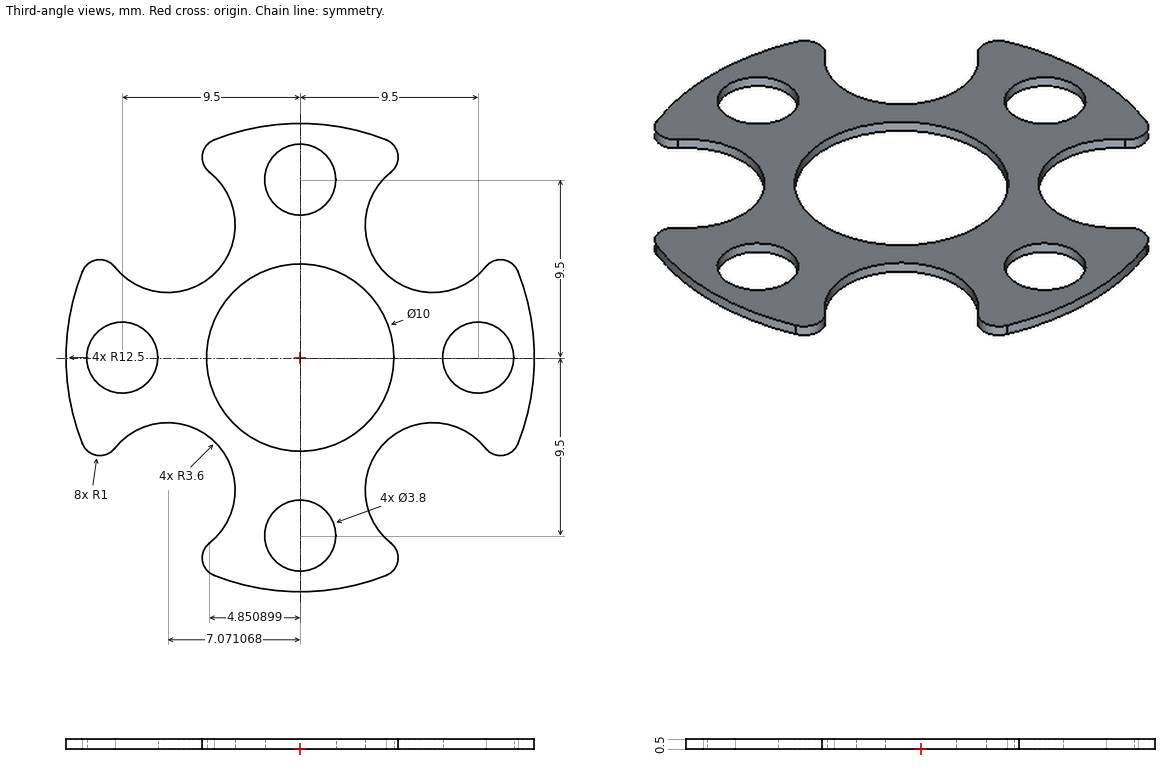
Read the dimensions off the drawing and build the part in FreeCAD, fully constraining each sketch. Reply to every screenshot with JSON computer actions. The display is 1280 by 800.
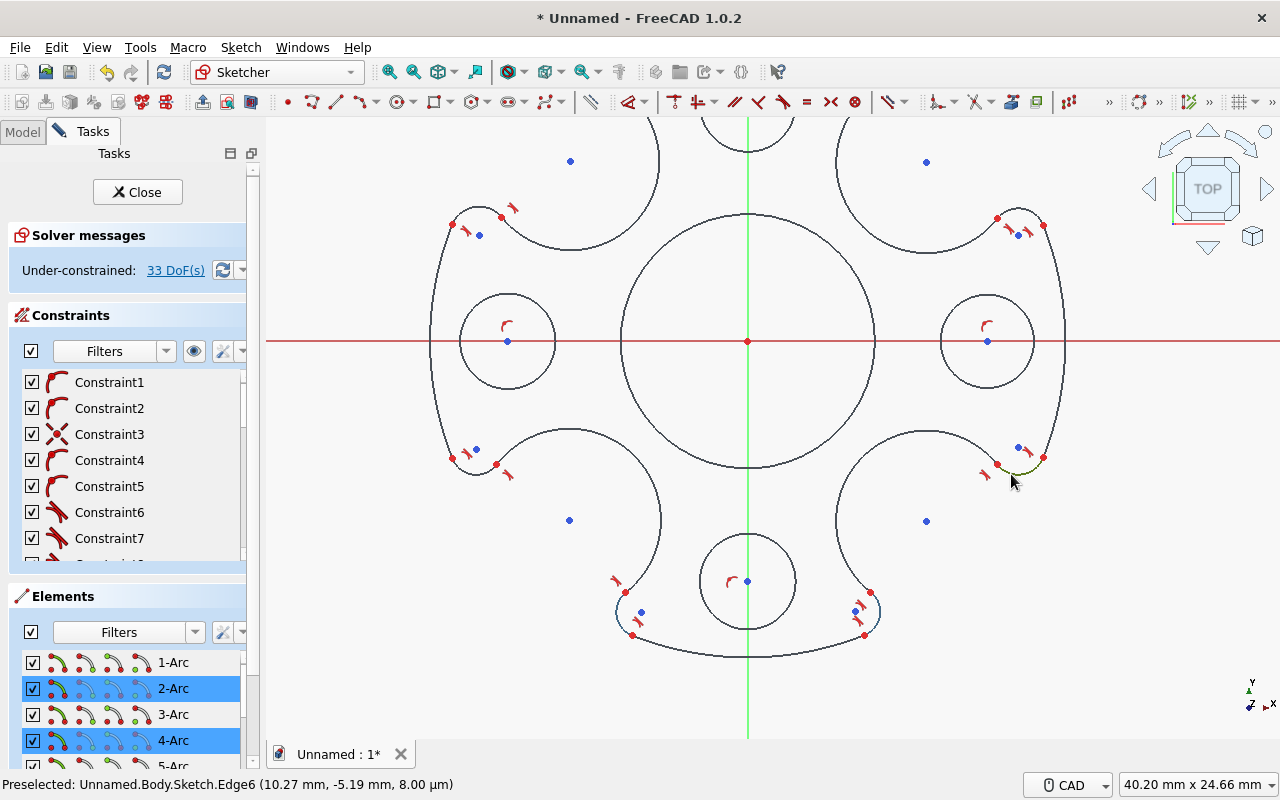
{"action": "left_click", "coordinate": [1033, 213]}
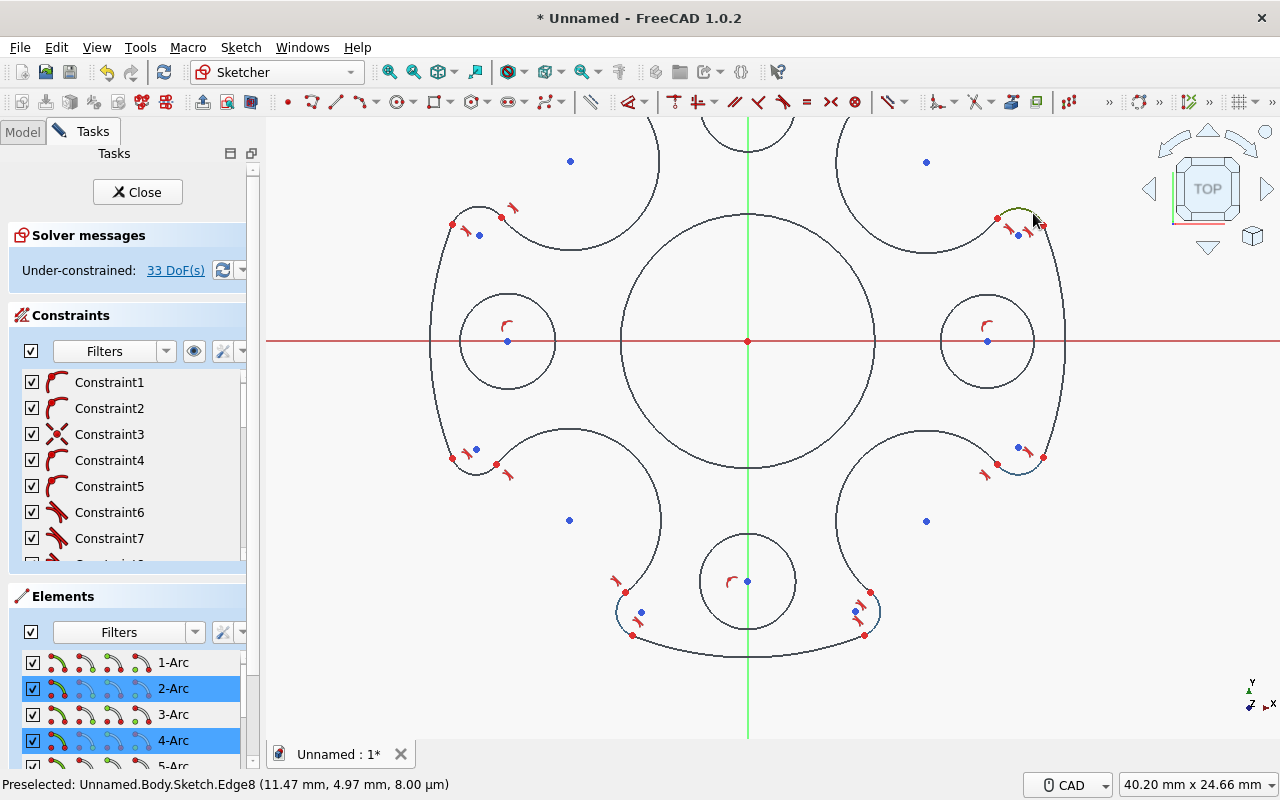
{"action": "scroll", "coordinate": [617, 604], "scroll_direction": "down", "scroll_amount": 2}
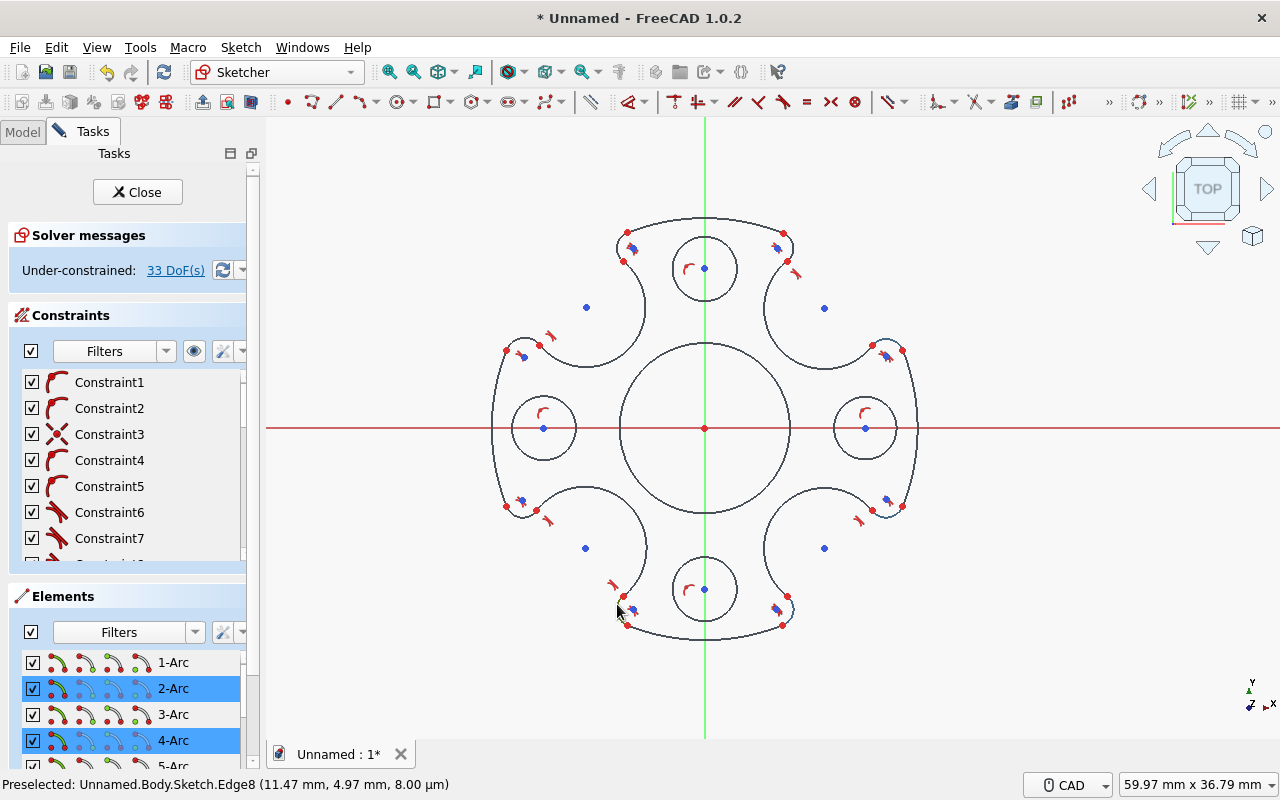
{"action": "scroll", "coordinate": [793, 253], "scroll_direction": "up", "scroll_amount": 2}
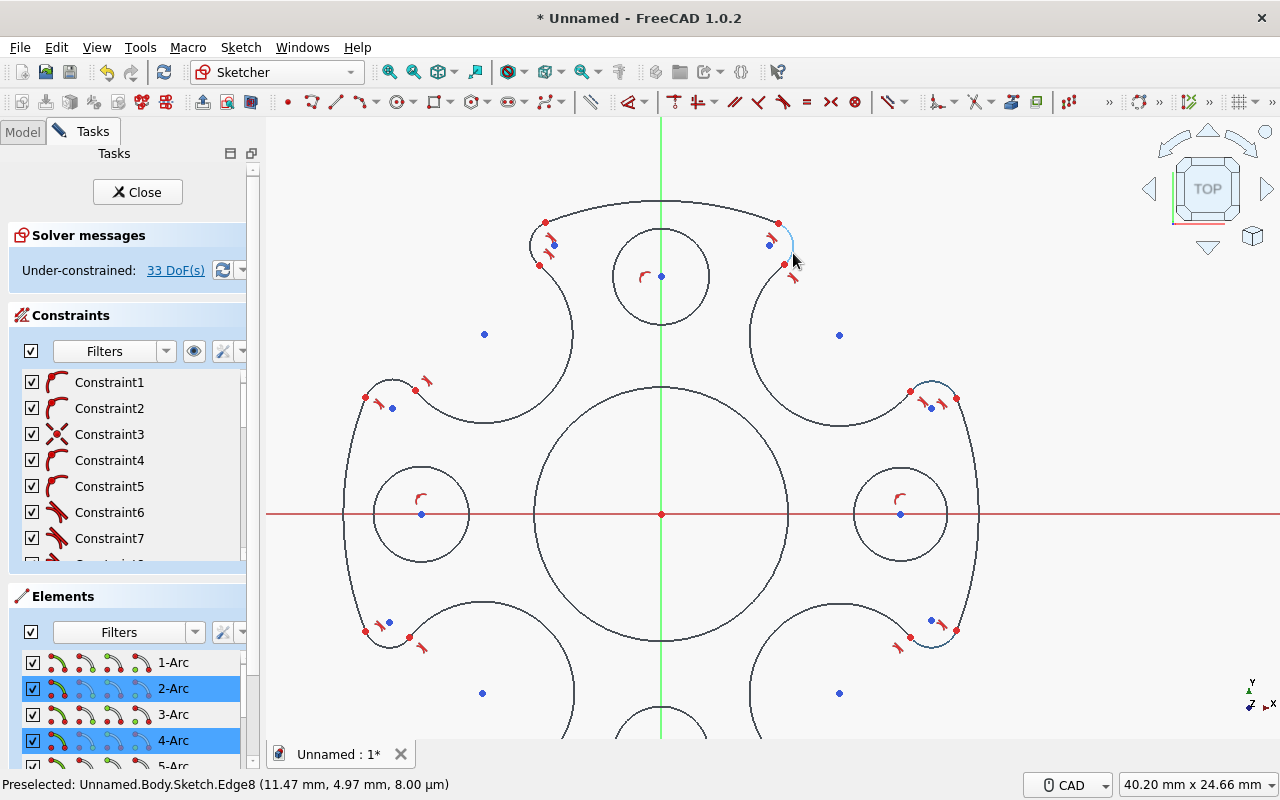
{"action": "left_click", "coordinate": [792, 253]}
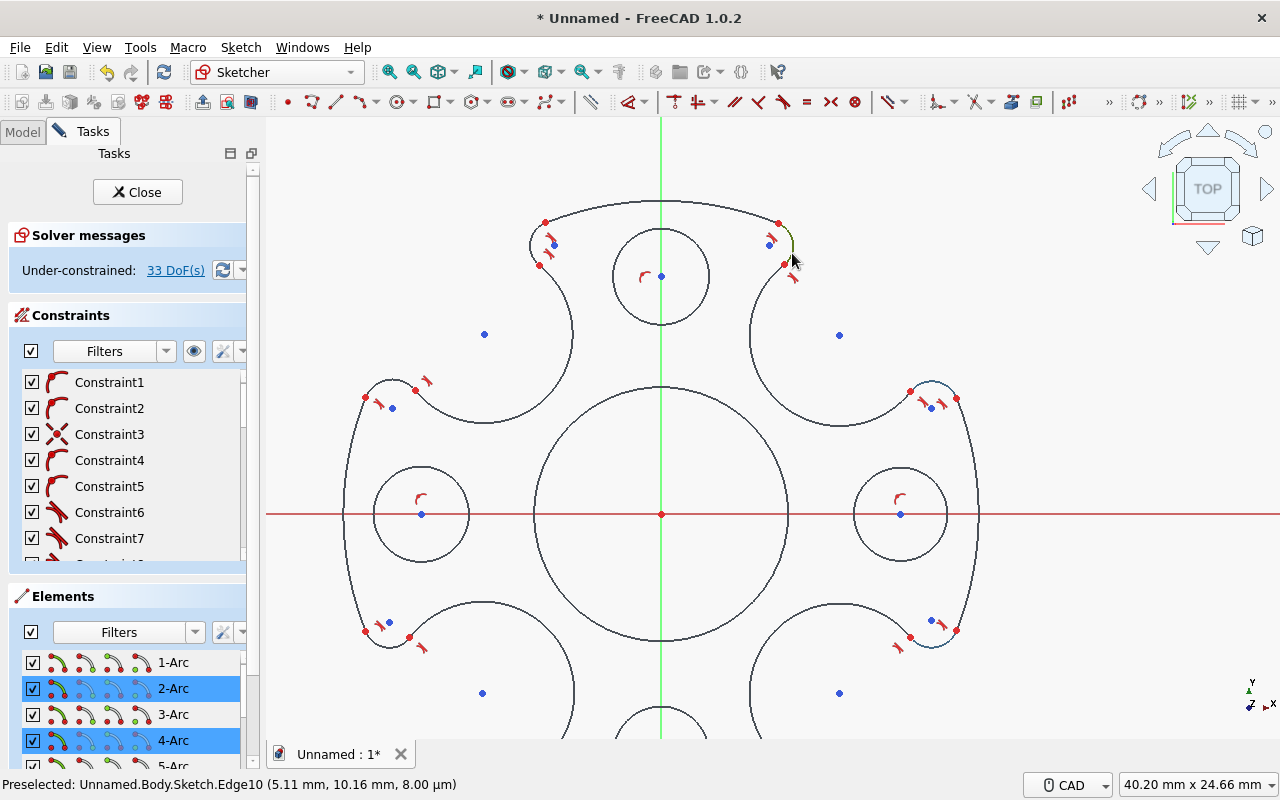
{"action": "left_click", "coordinate": [534, 233]}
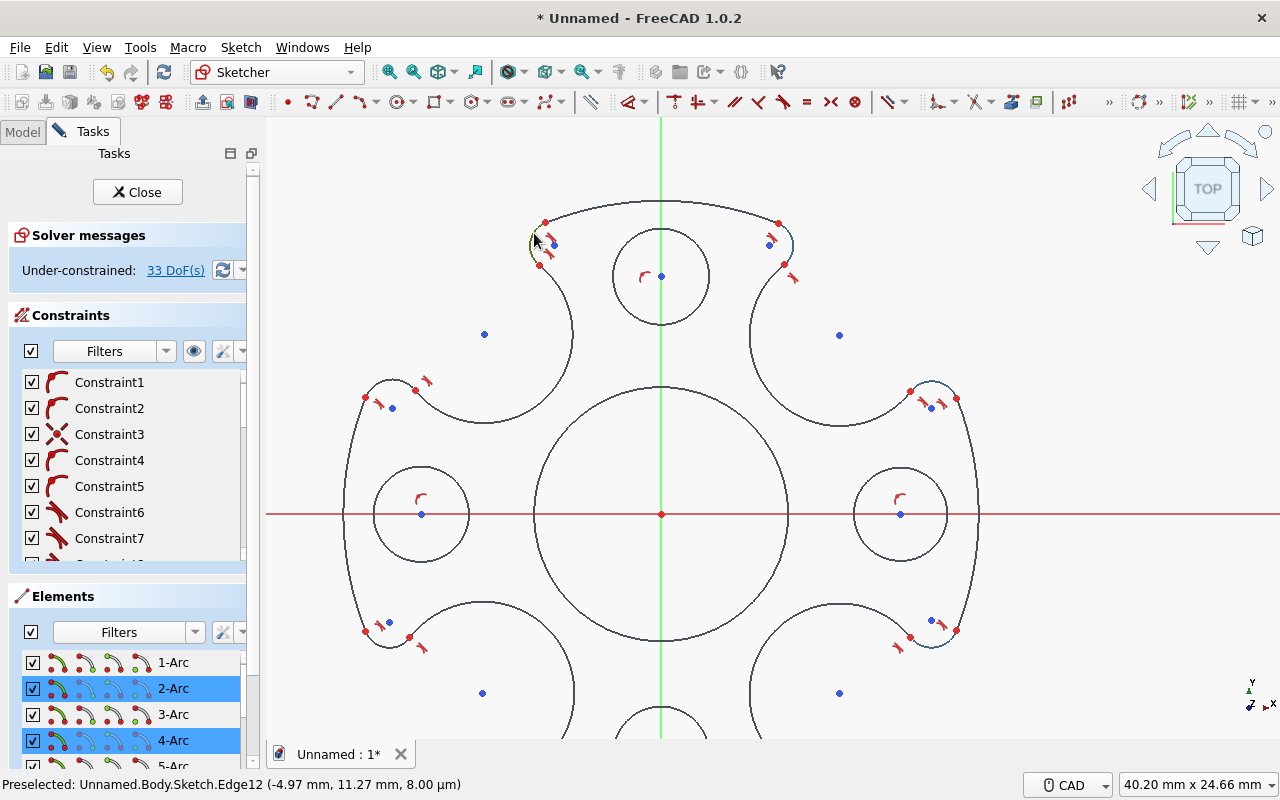
{"action": "left_click", "coordinate": [400, 381]}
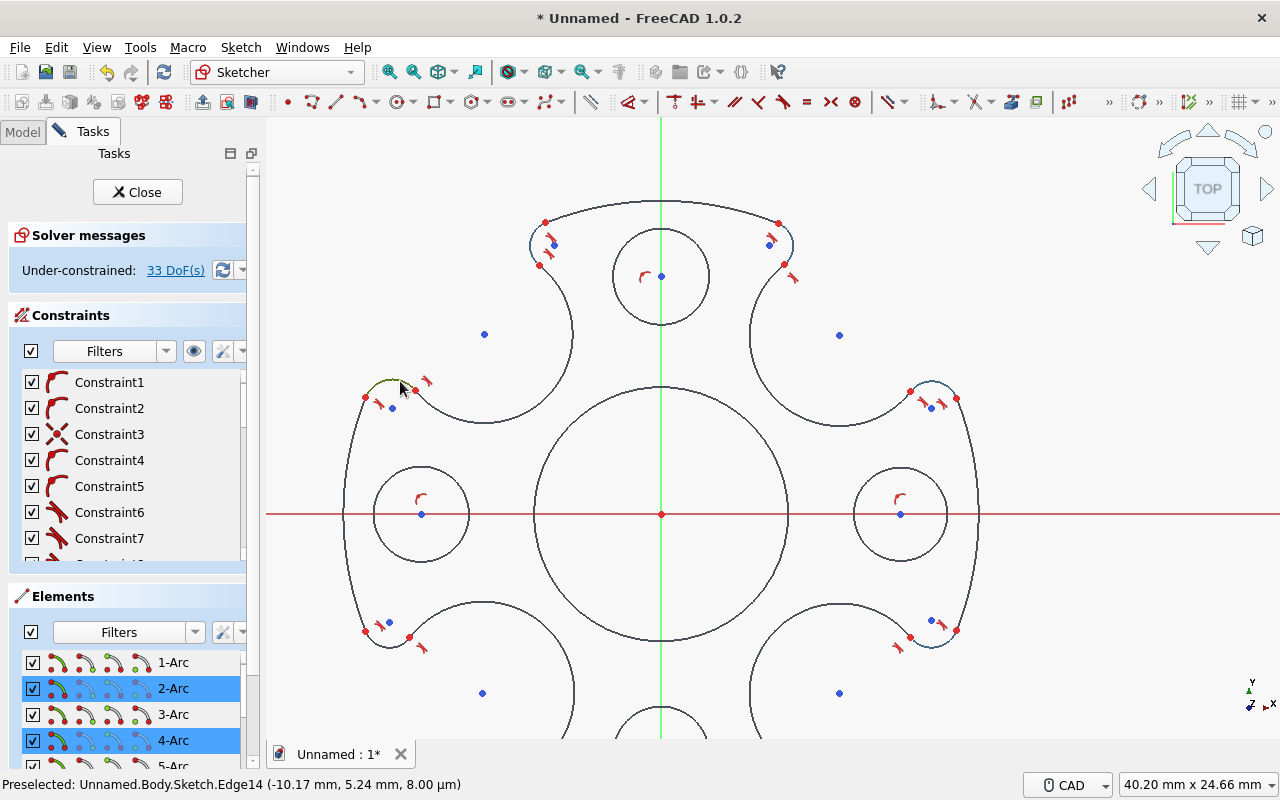
{"action": "left_click", "coordinate": [376, 644]}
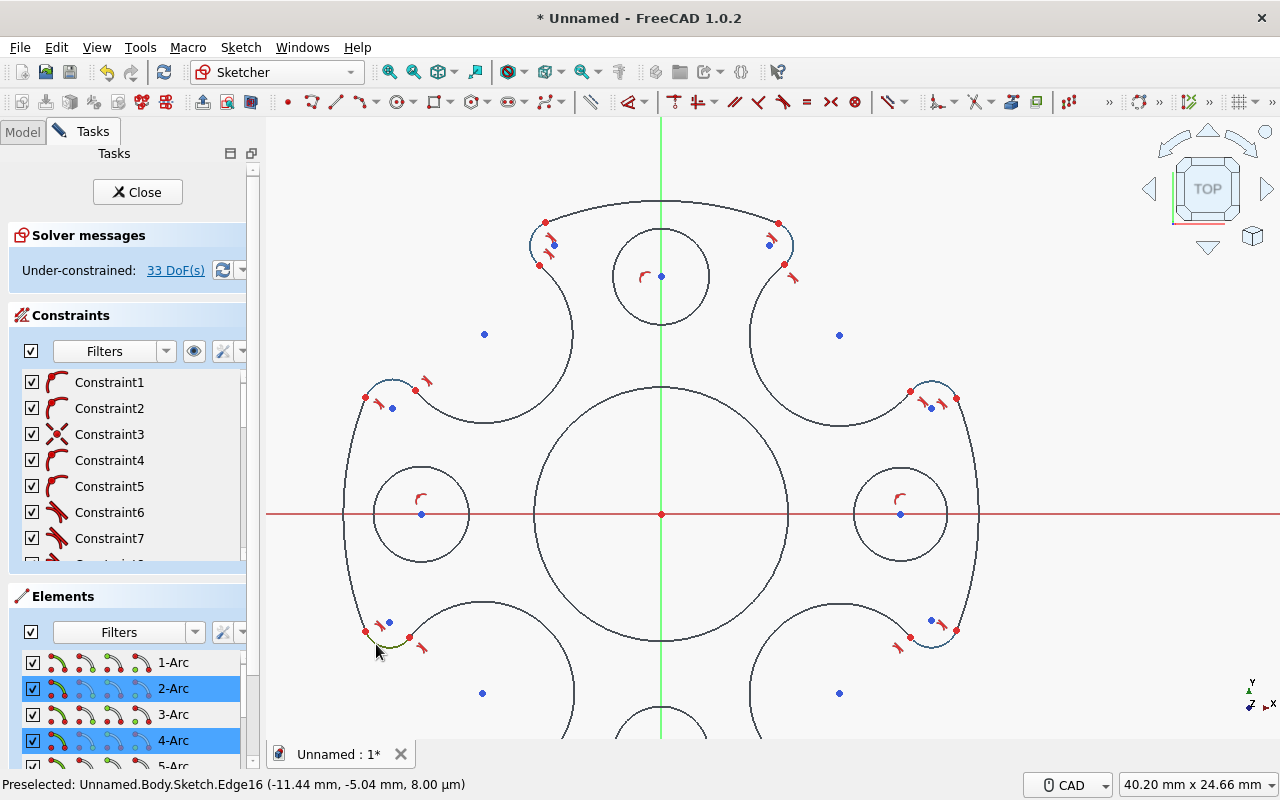
{"action": "key", "text": "e"}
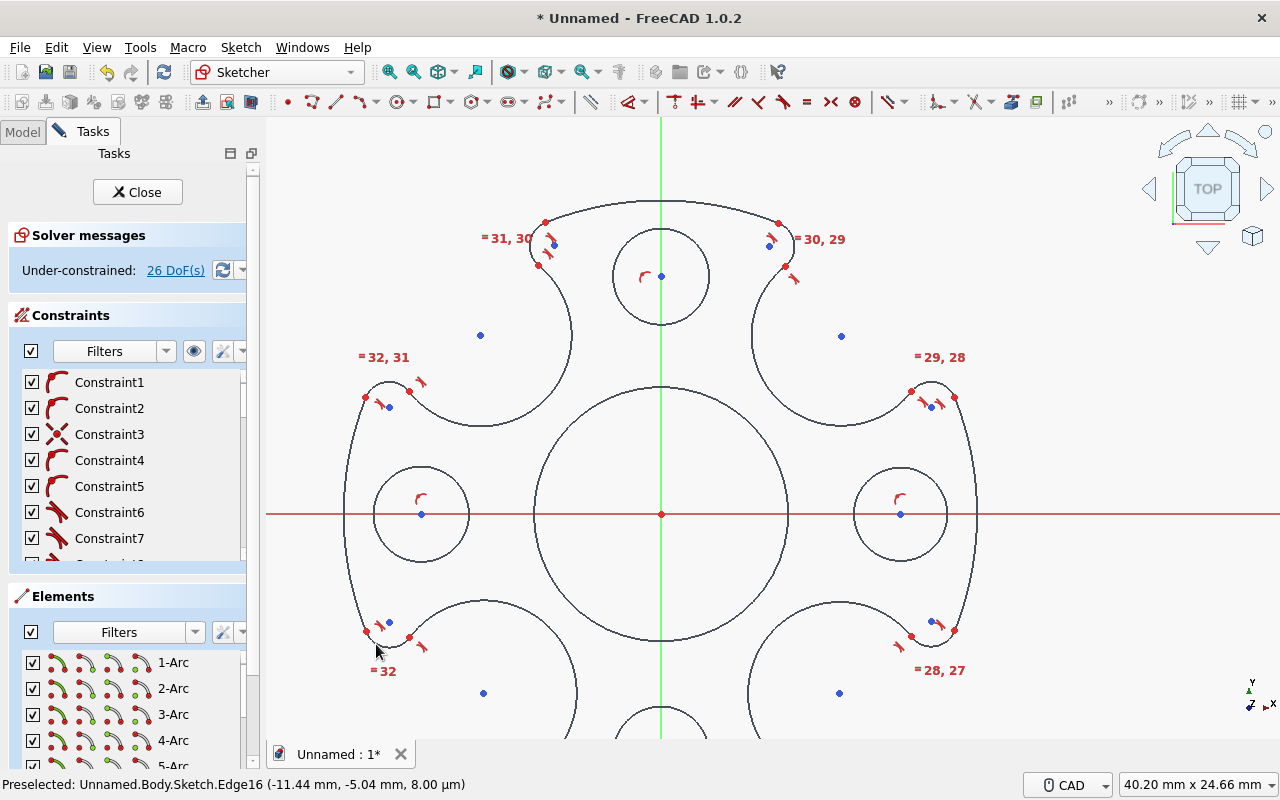
{"action": "left_click", "coordinate": [576, 683]}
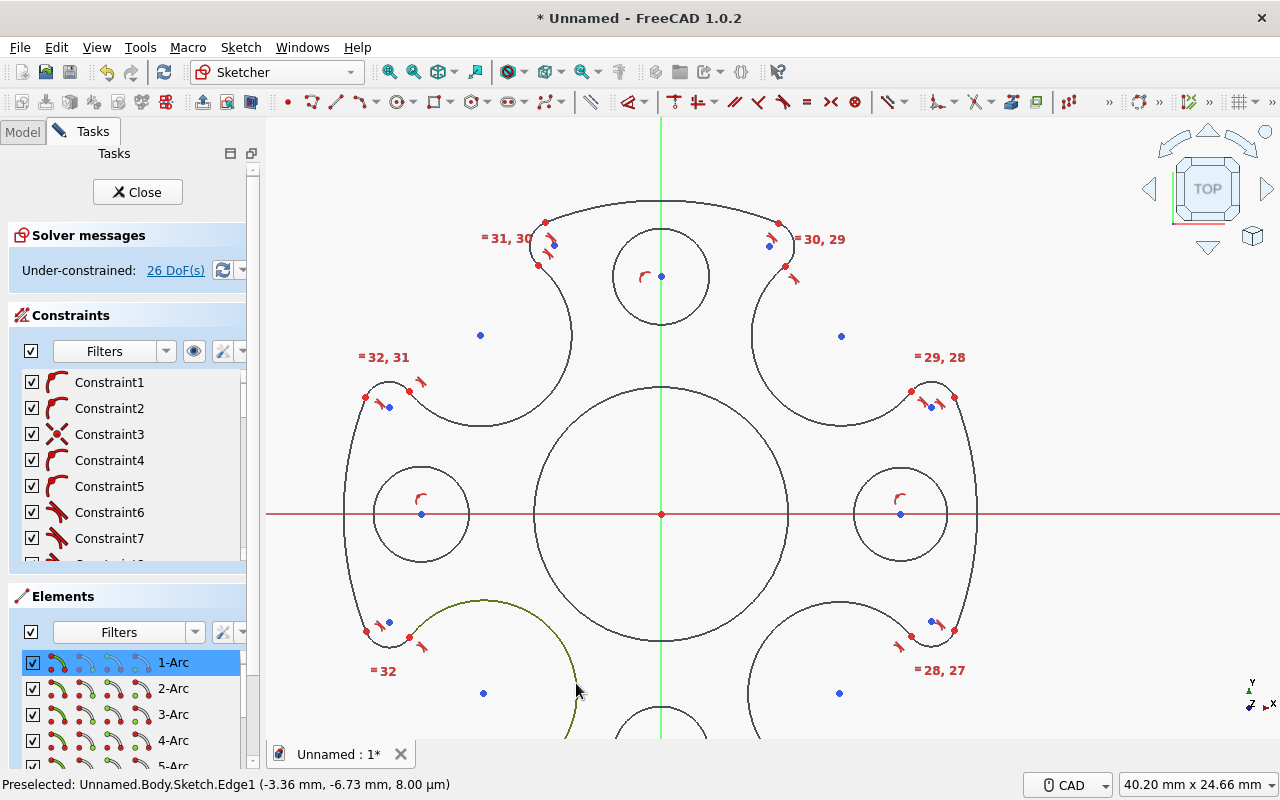
{"action": "left_click", "coordinate": [829, 603]}